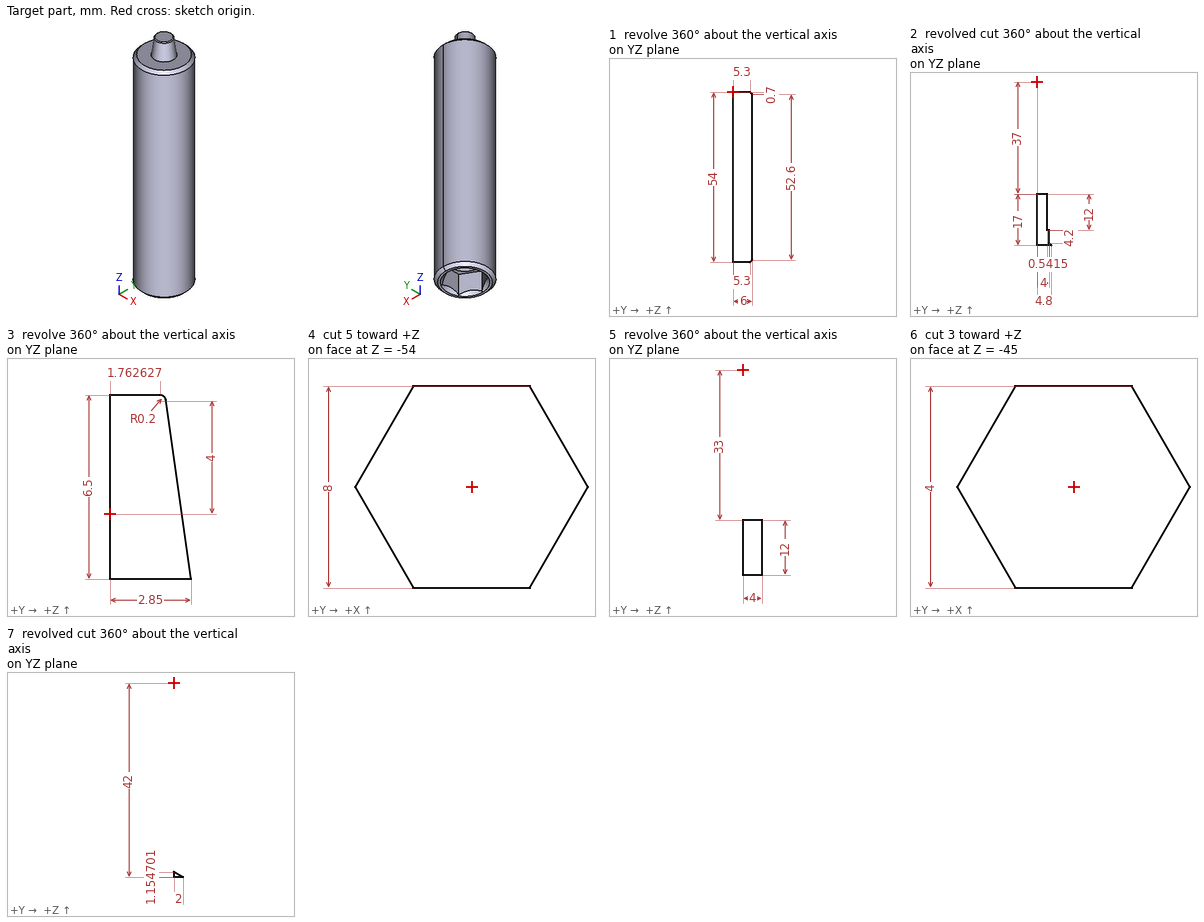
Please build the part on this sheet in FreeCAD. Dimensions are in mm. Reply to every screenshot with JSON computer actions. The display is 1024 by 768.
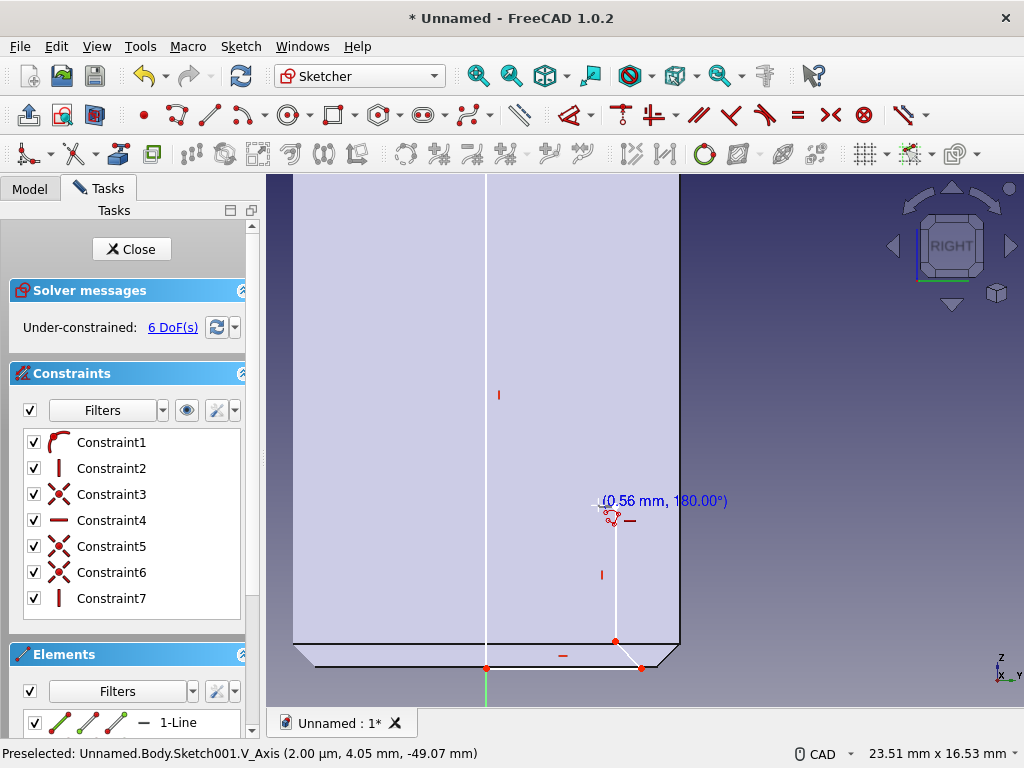
{"action": "left_click", "coordinate": [598, 505]}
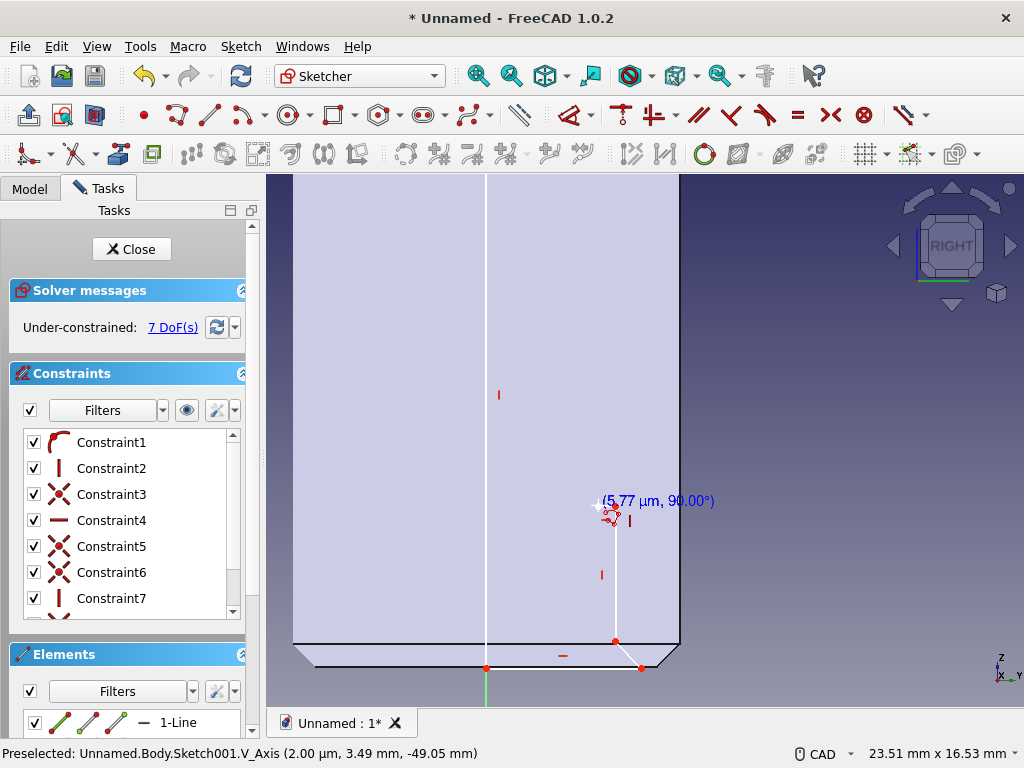
{"action": "scroll", "coordinate": [602, 538], "scroll_direction": "down", "scroll_amount": 2}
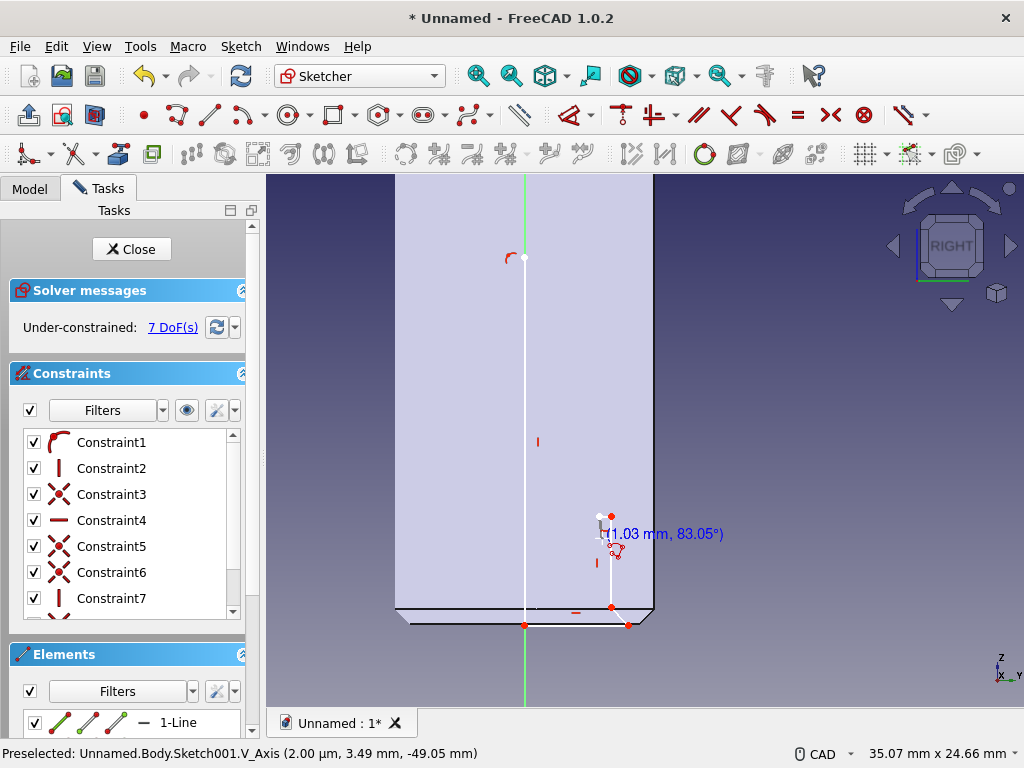
{"action": "left_click", "coordinate": [599, 257]}
{"action": "left_click", "coordinate": [525, 258]}
{"action": "key", "text": "Escape"}
{"action": "key", "text": "Escape"}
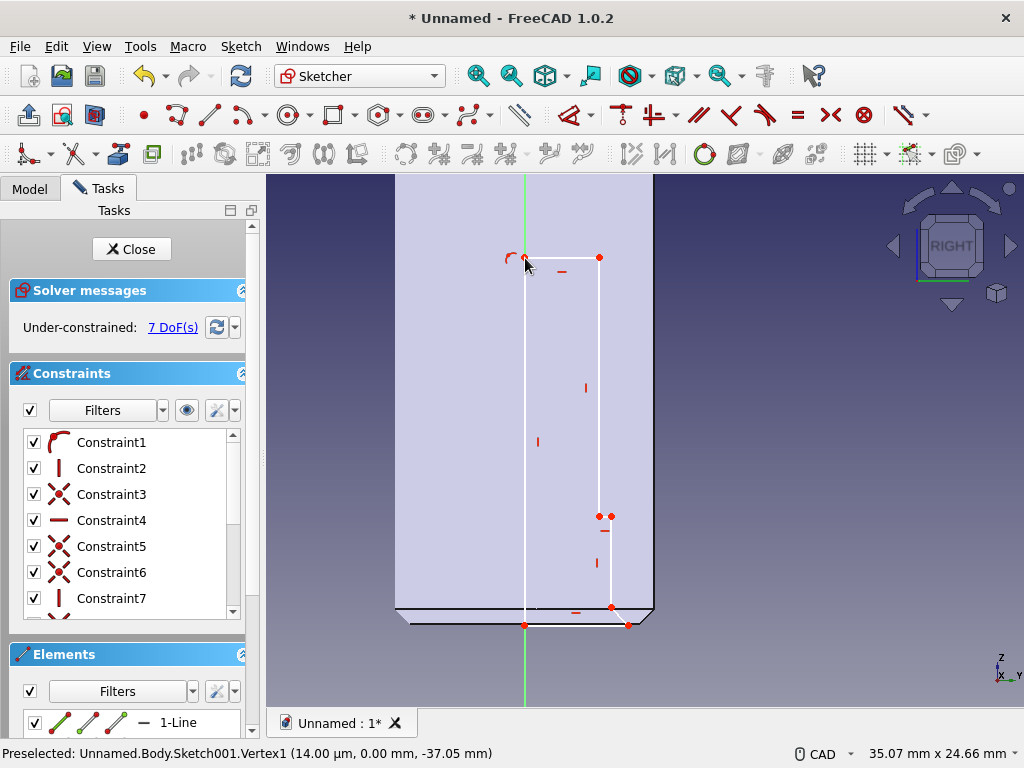
{"action": "left_click", "coordinate": [568, 116]}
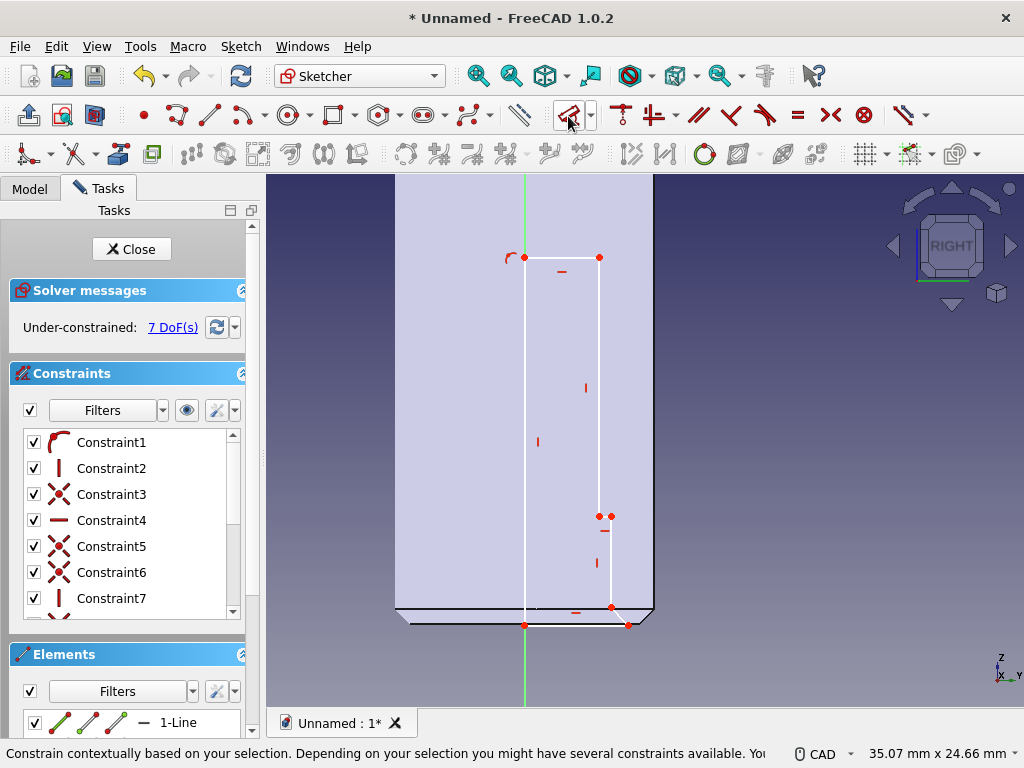
{"action": "left_click", "coordinate": [525, 368]}
{"action": "left_click", "coordinate": [491, 442]}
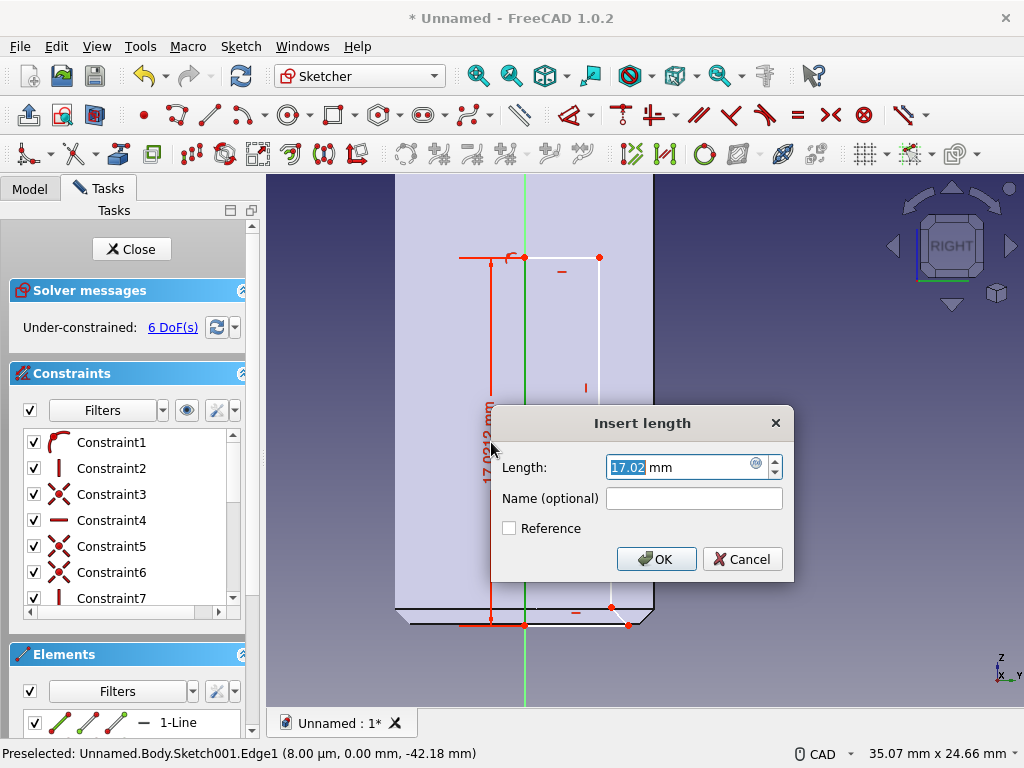
{"action": "type", "text": "17"}
{"action": "key", "text": "Return"}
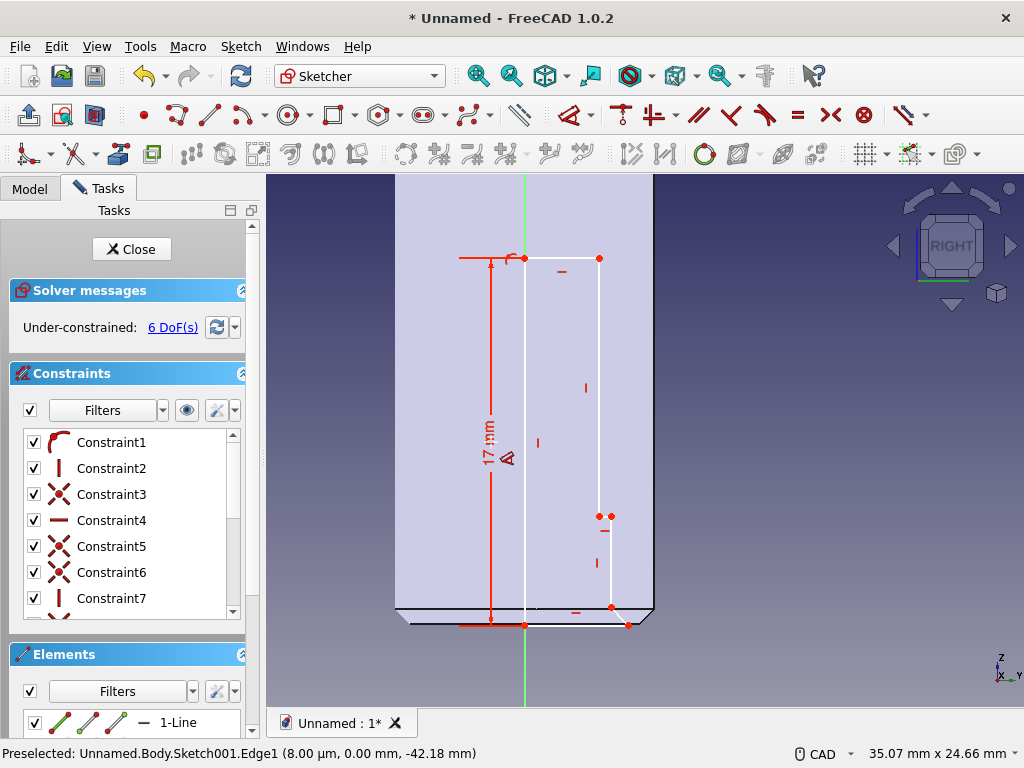
{"action": "left_click", "coordinate": [599, 439]}
{"action": "left_click", "coordinate": [633, 388]}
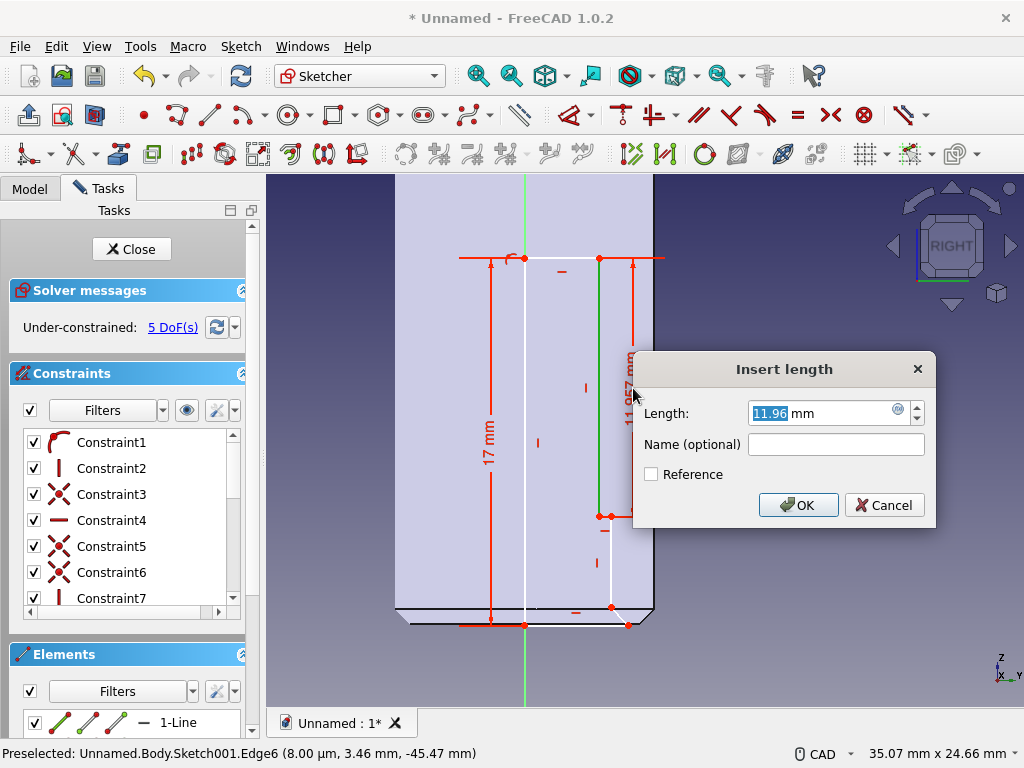
{"action": "type", "text": "12"}
{"action": "key", "text": "Return"}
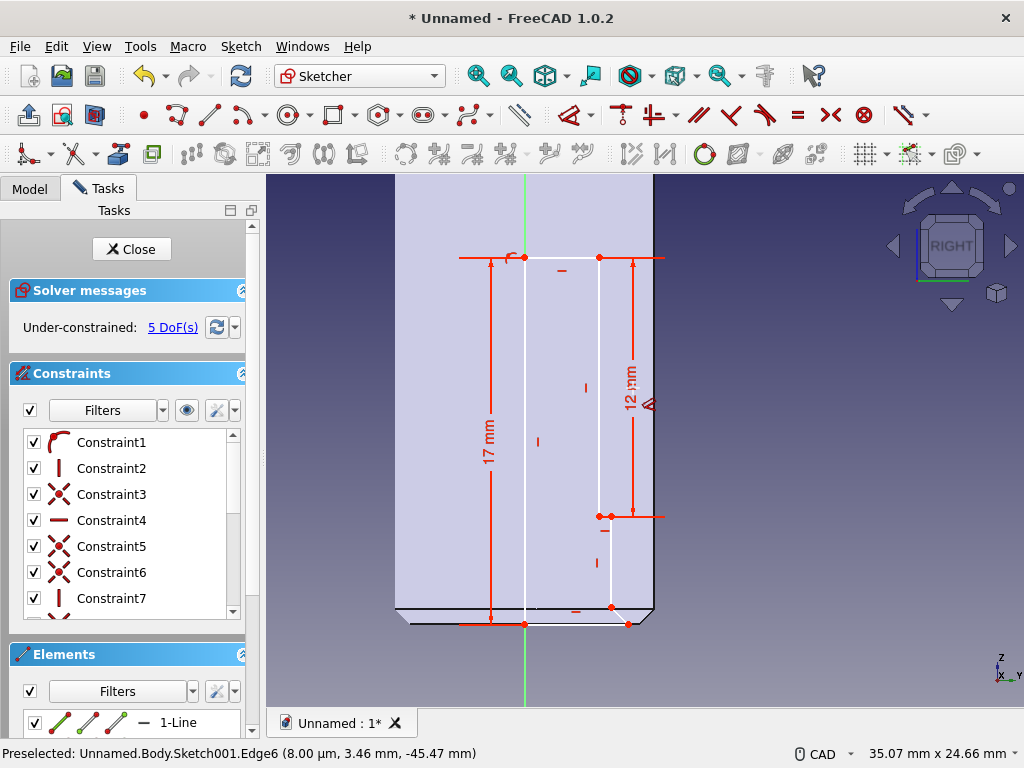
{"action": "left_click", "coordinate": [611, 608]}
{"action": "left_click", "coordinate": [568, 642]}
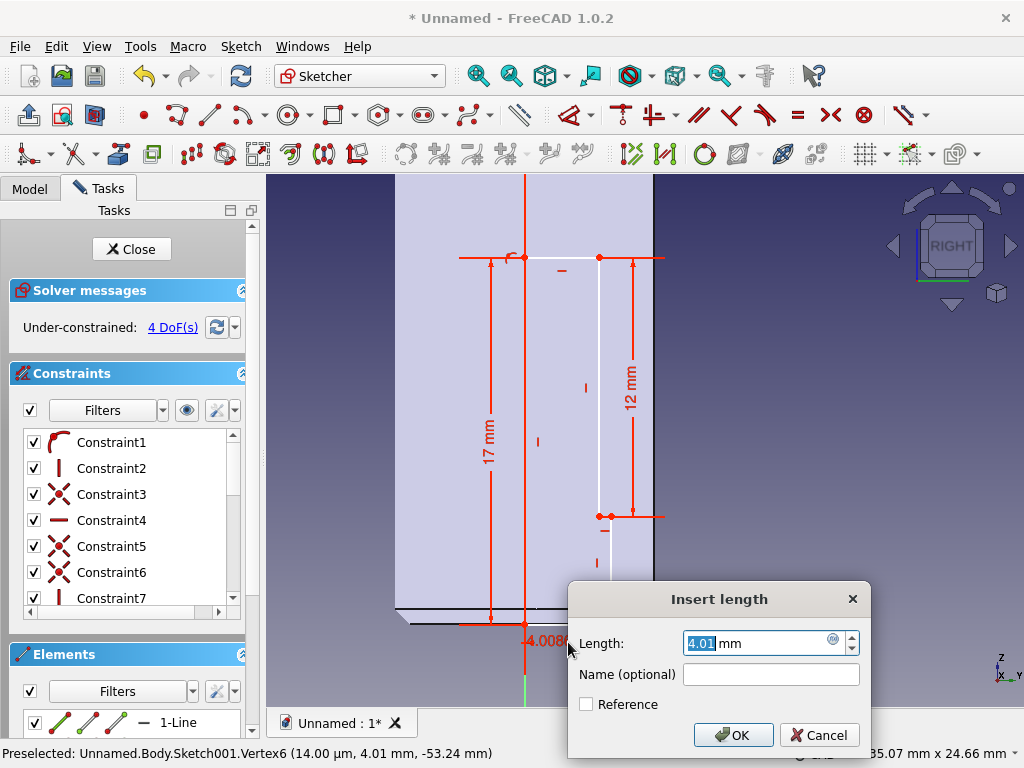
{"action": "type", "text": "4"}
{"action": "key", "text": "Return"}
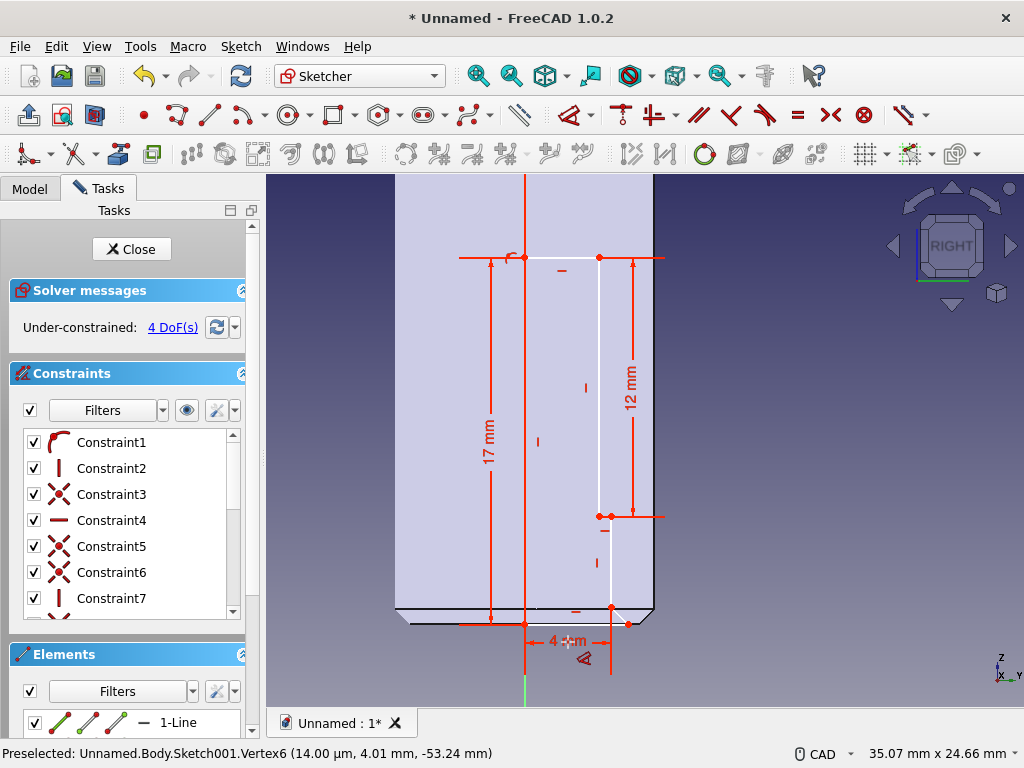
{"action": "left_click", "coordinate": [556, 625]}
{"action": "left_click", "coordinate": [576, 591]}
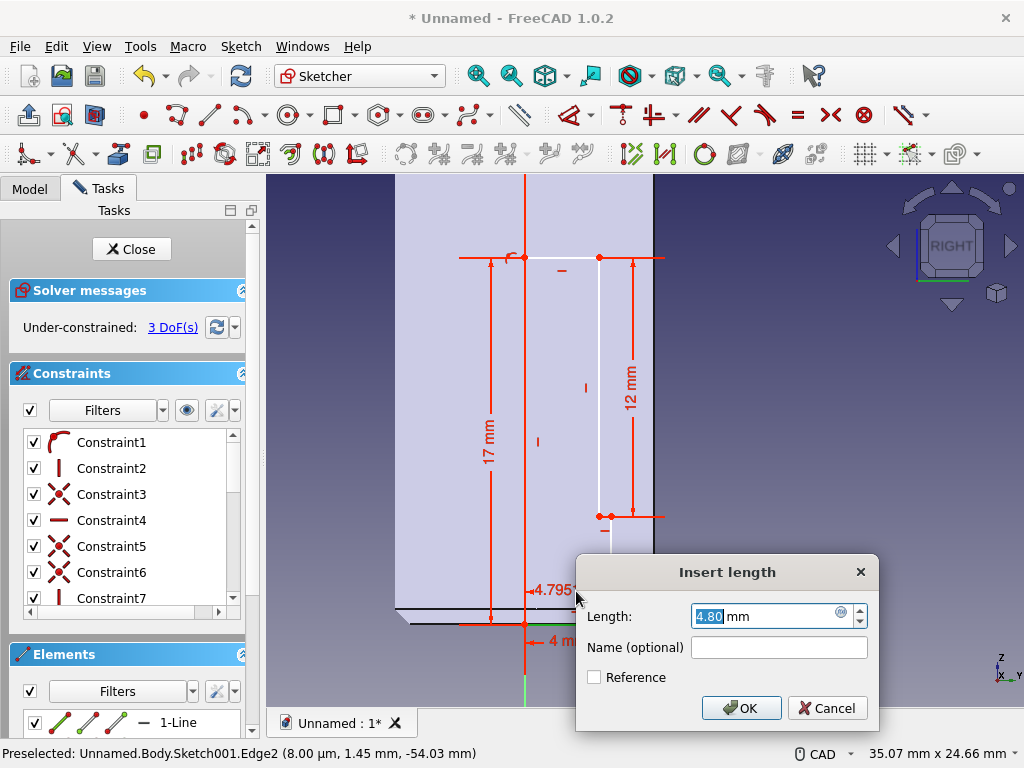
{"action": "type", "text": "4.8"}
{"action": "key", "text": "Return"}